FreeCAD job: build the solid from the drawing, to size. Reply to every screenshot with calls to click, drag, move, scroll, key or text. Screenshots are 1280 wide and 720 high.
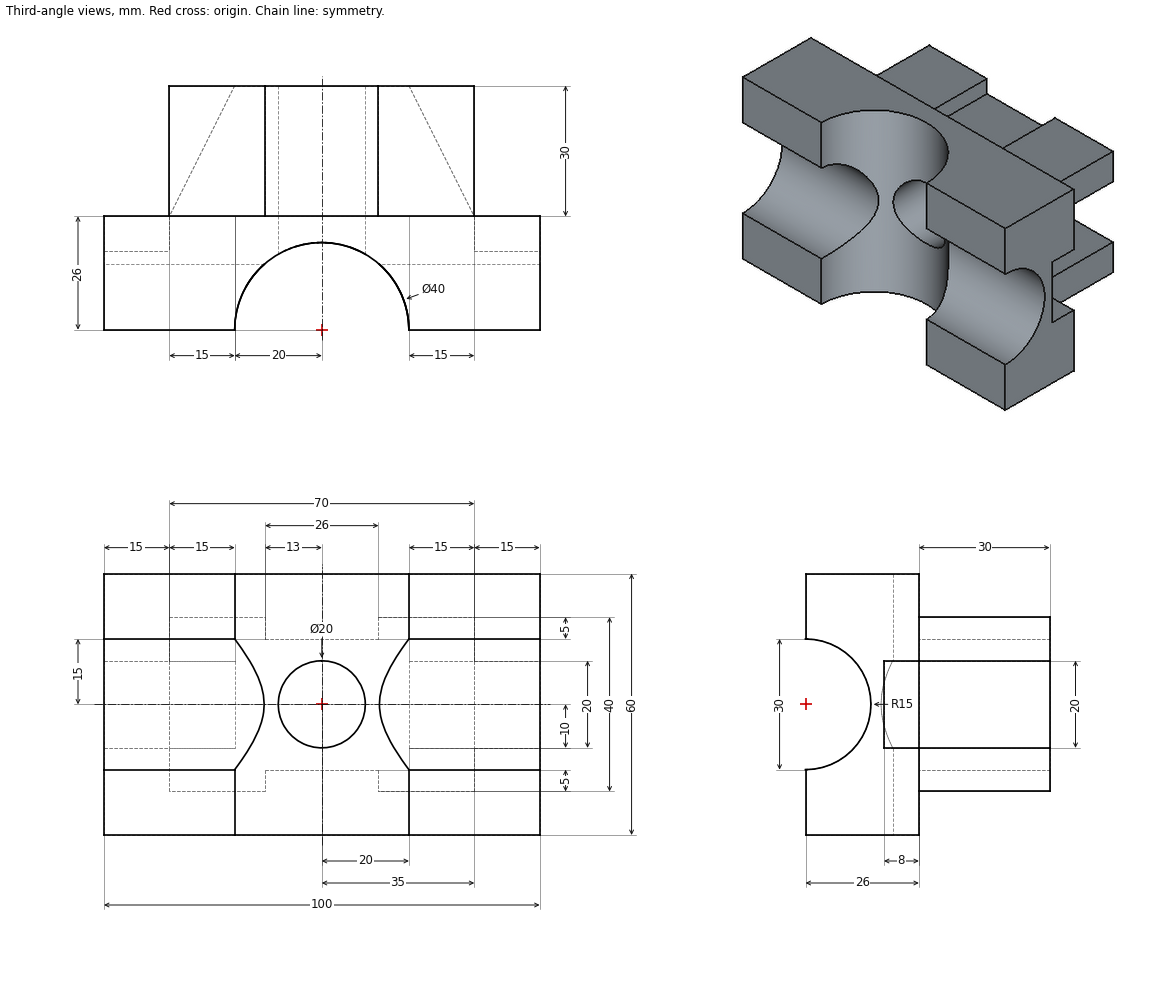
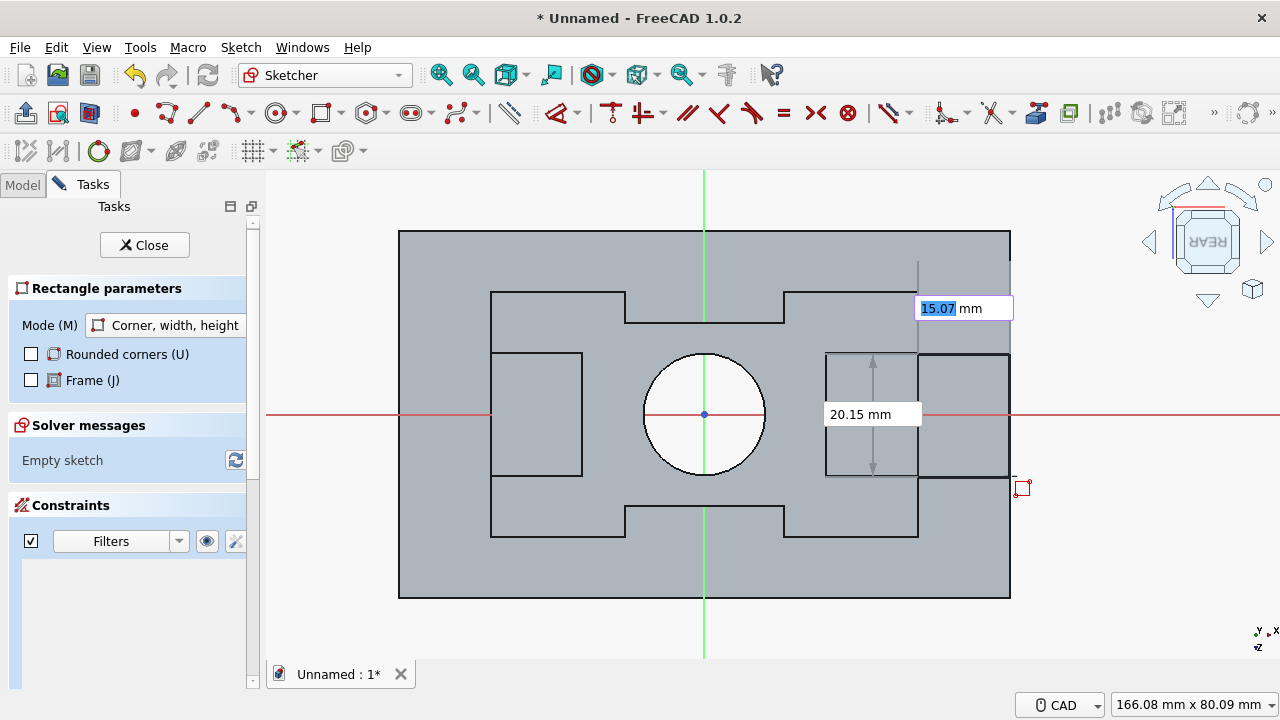
text(15)
key(Tab)
text(20)
key(Return)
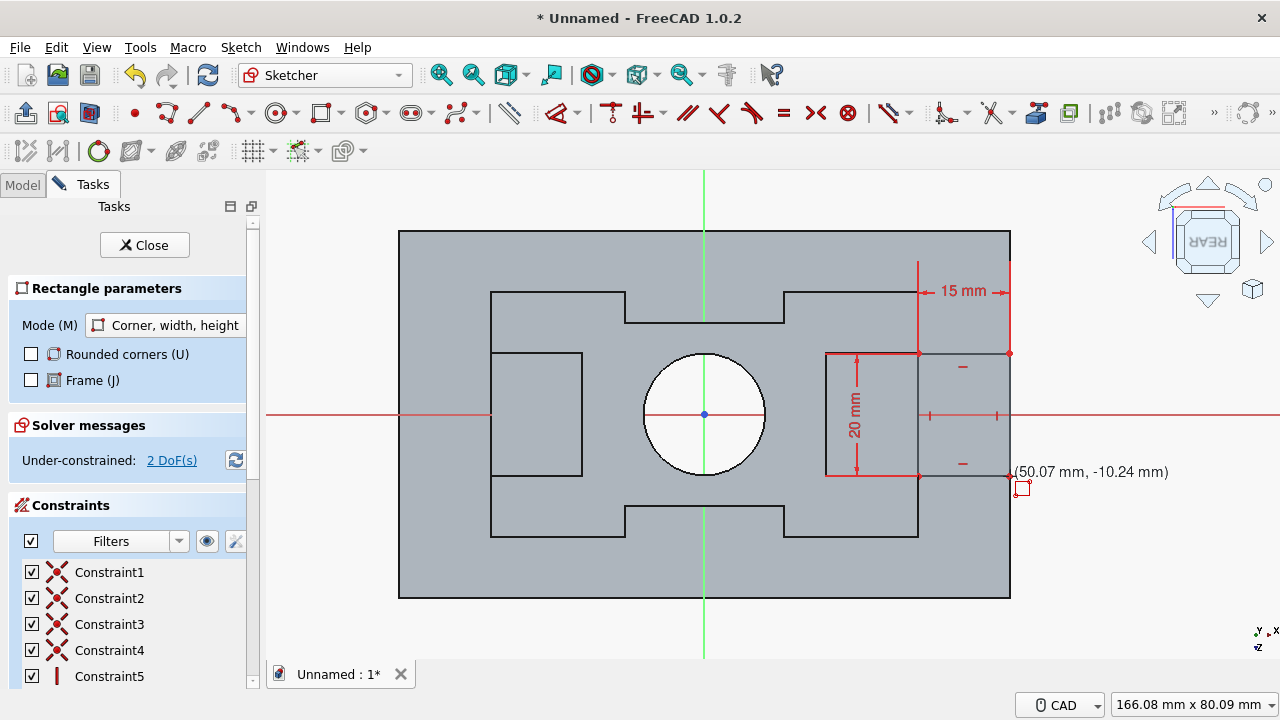
click(399, 353)
move(491, 476)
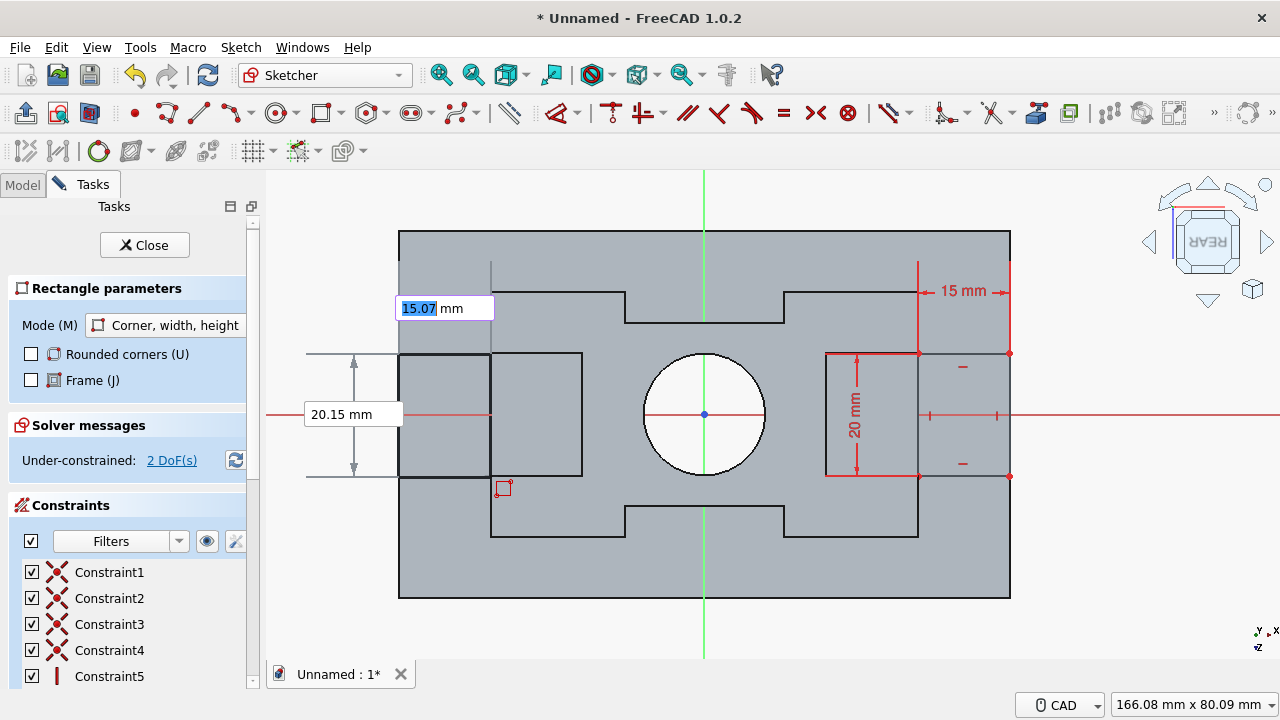
text(15)
key(Tab)
text(20)
key(Return)
key(Escape)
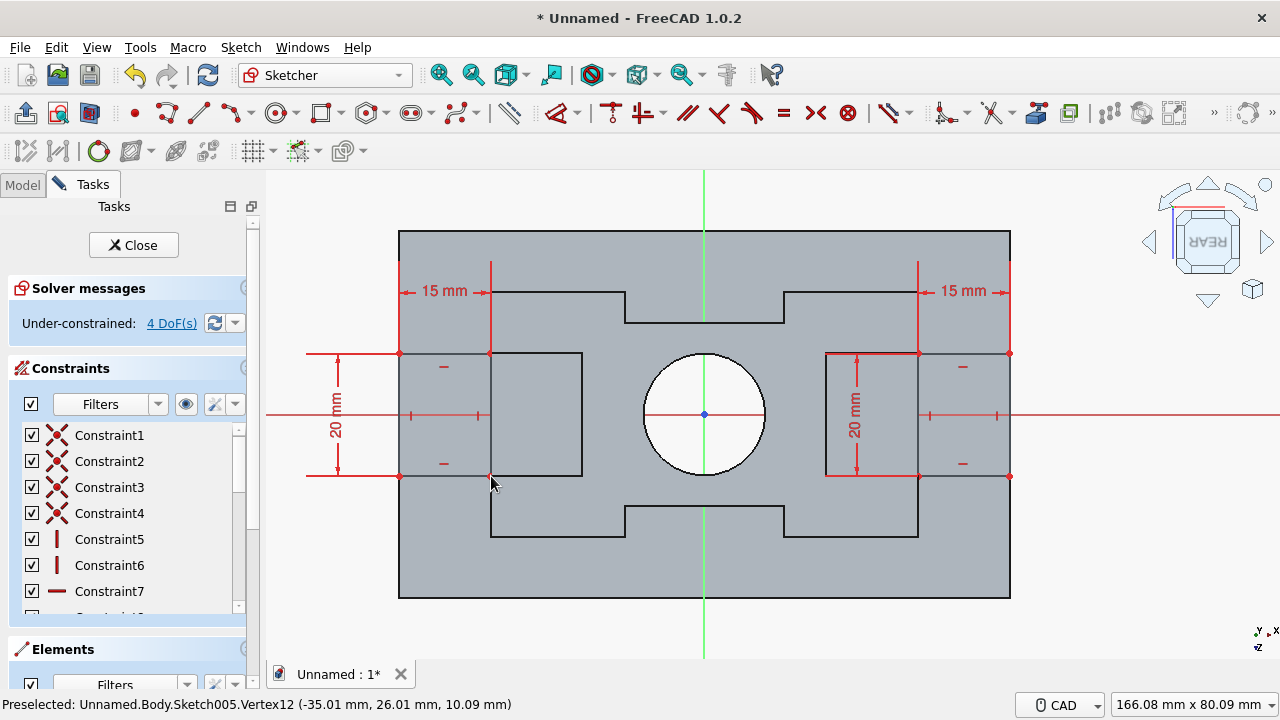
click(1010, 354)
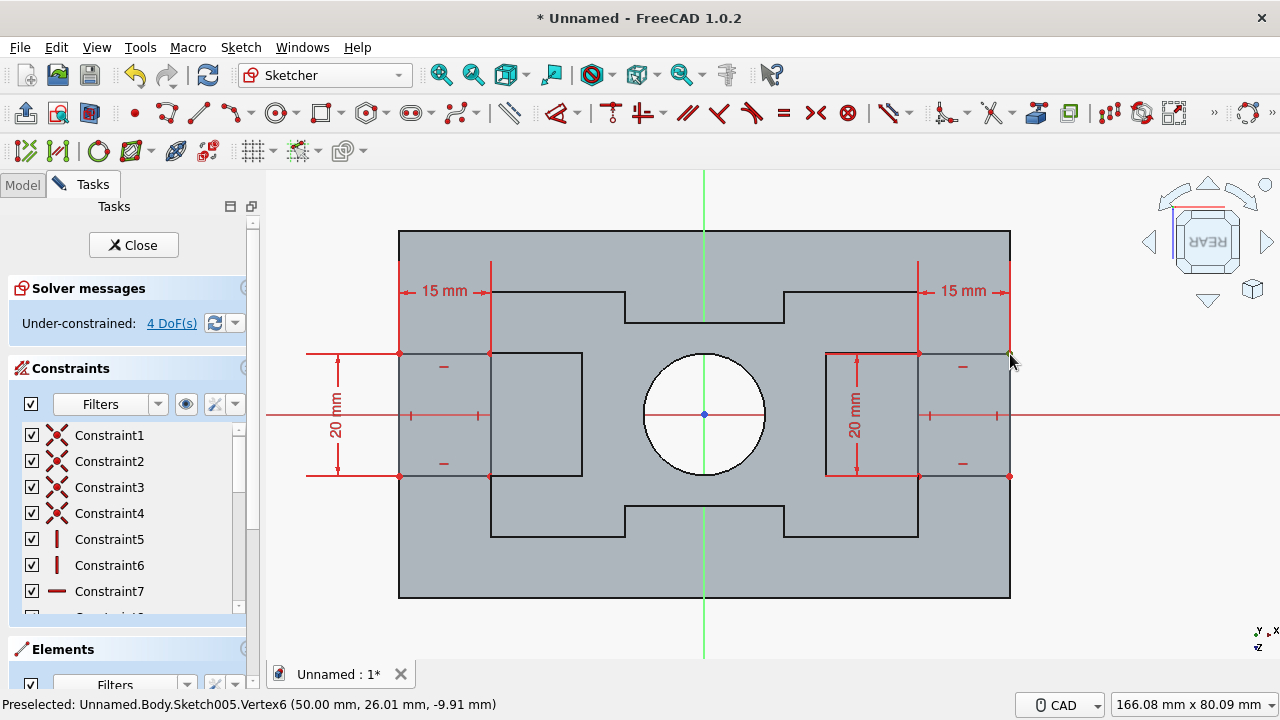
click(399, 354)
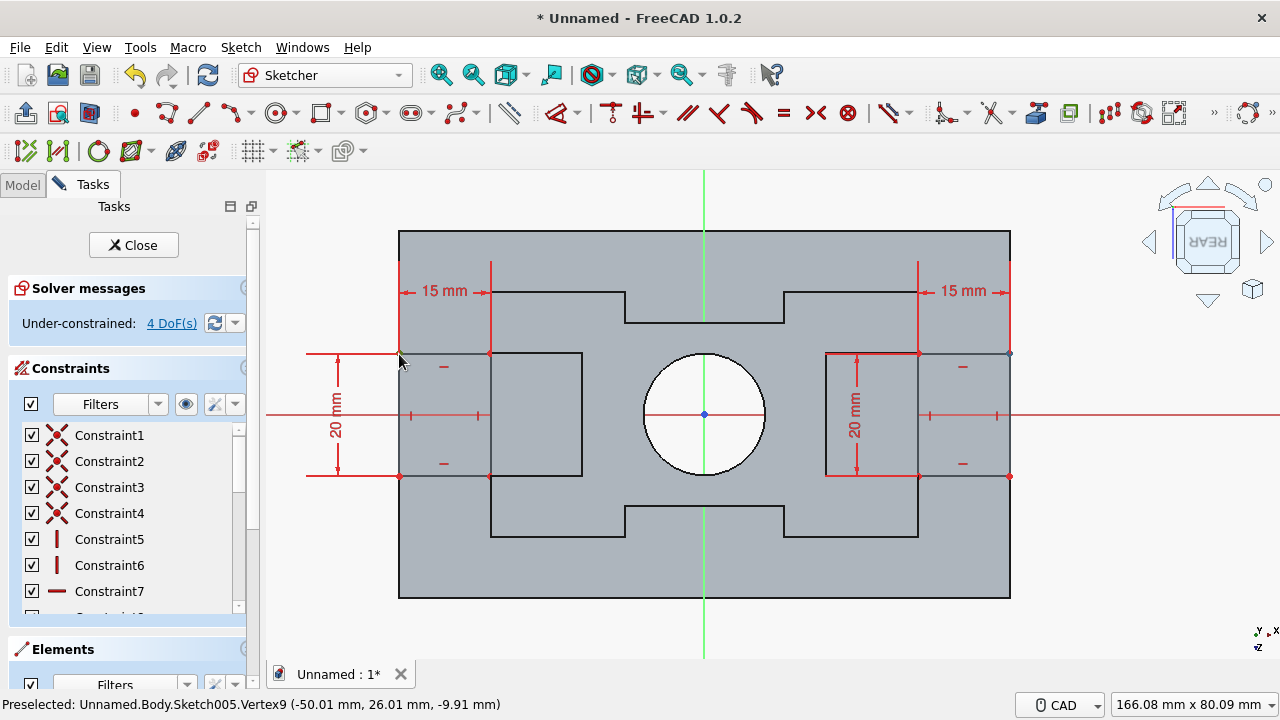
click(704, 600)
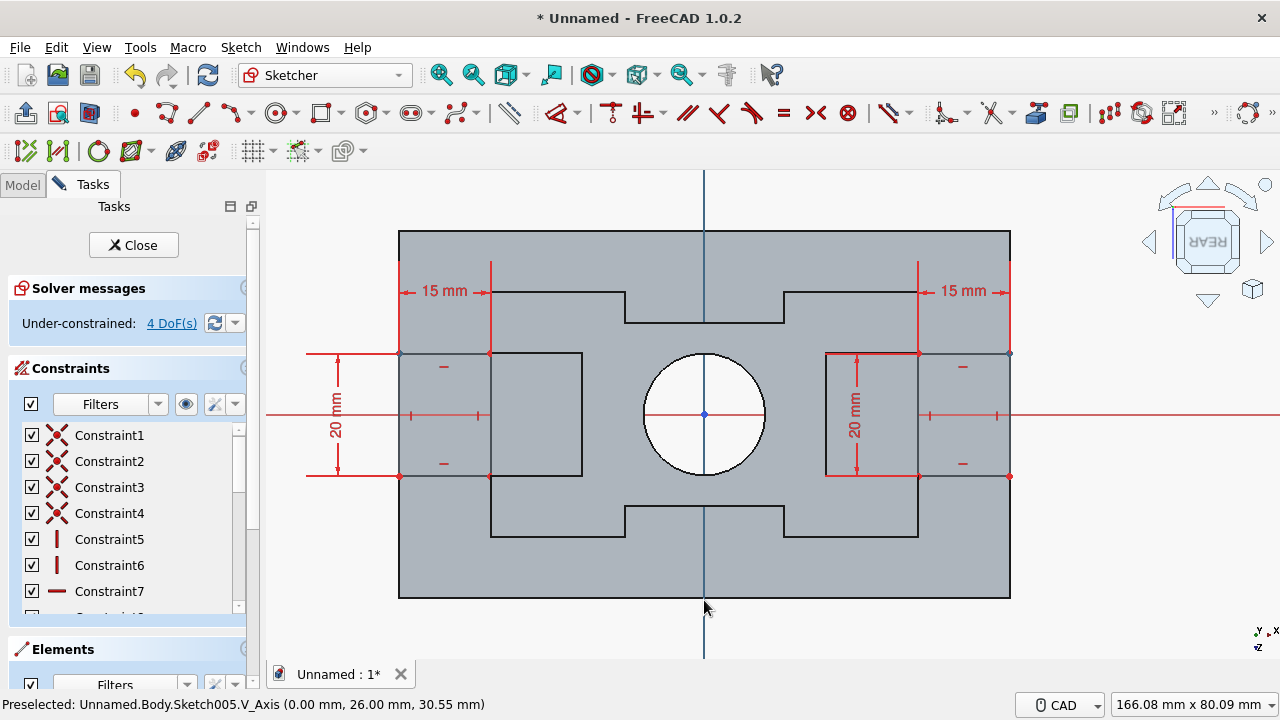
key(s)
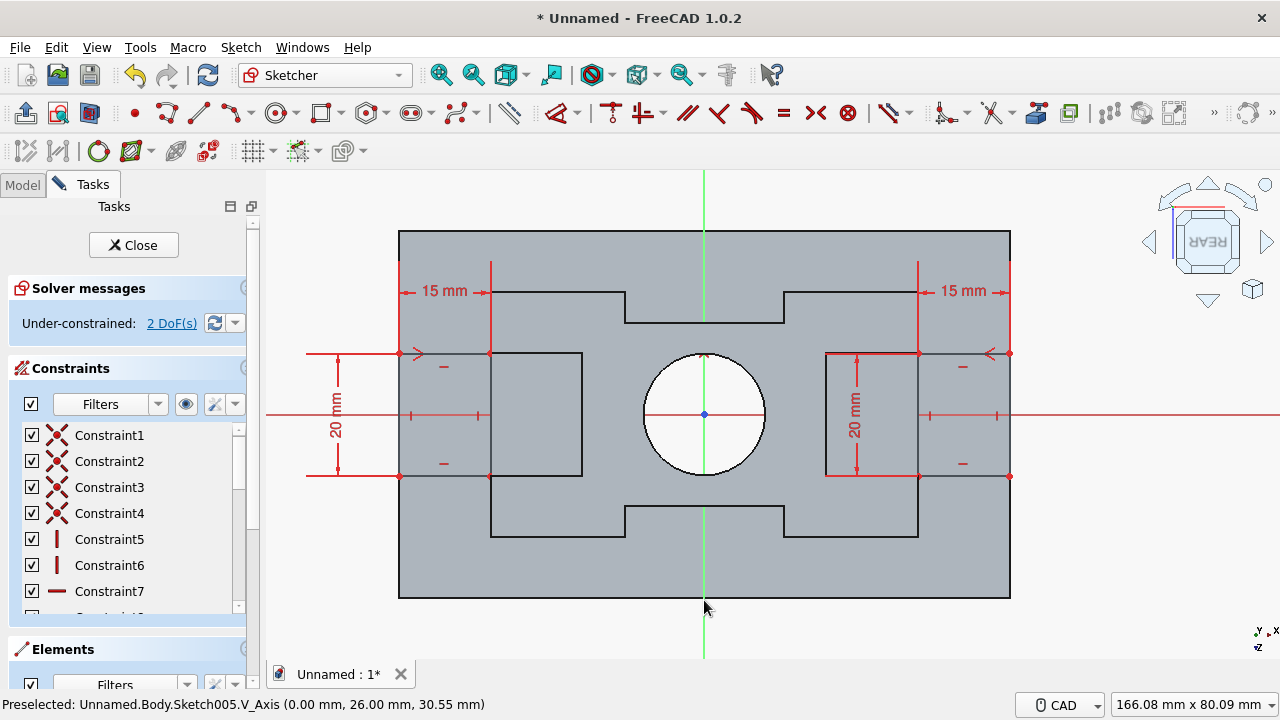
key(d)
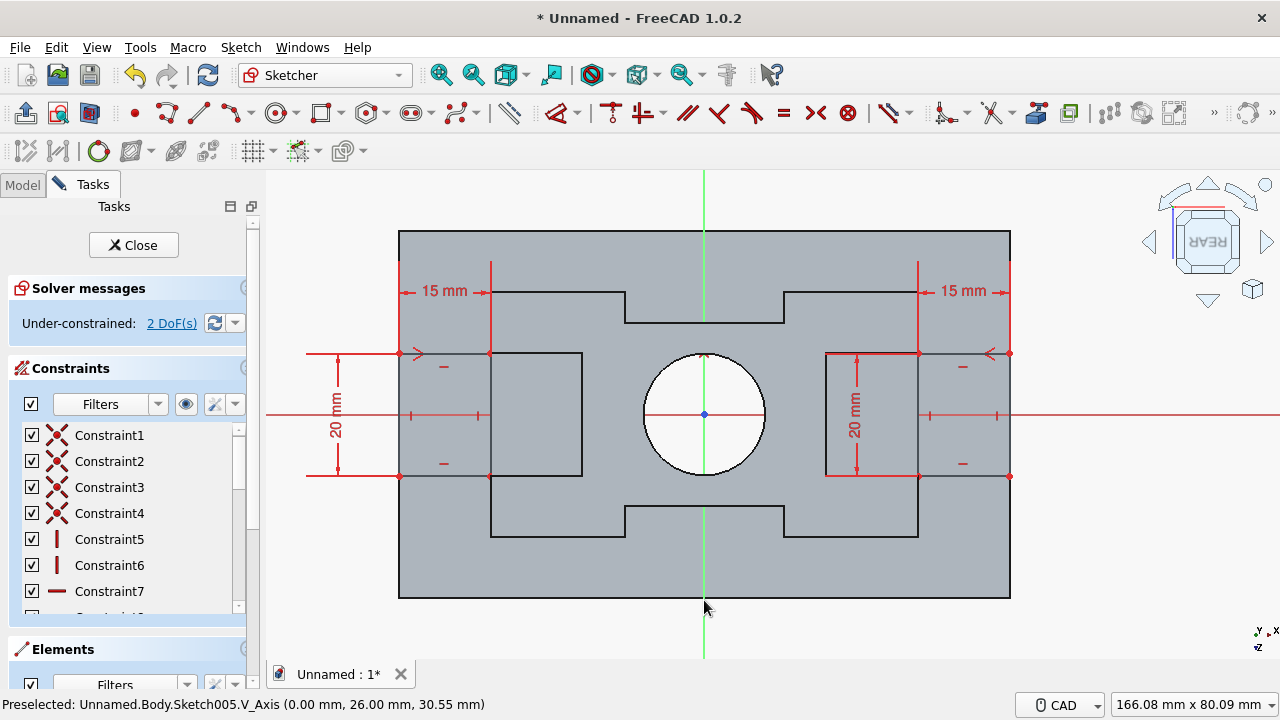
click(918, 354)
click(811, 320)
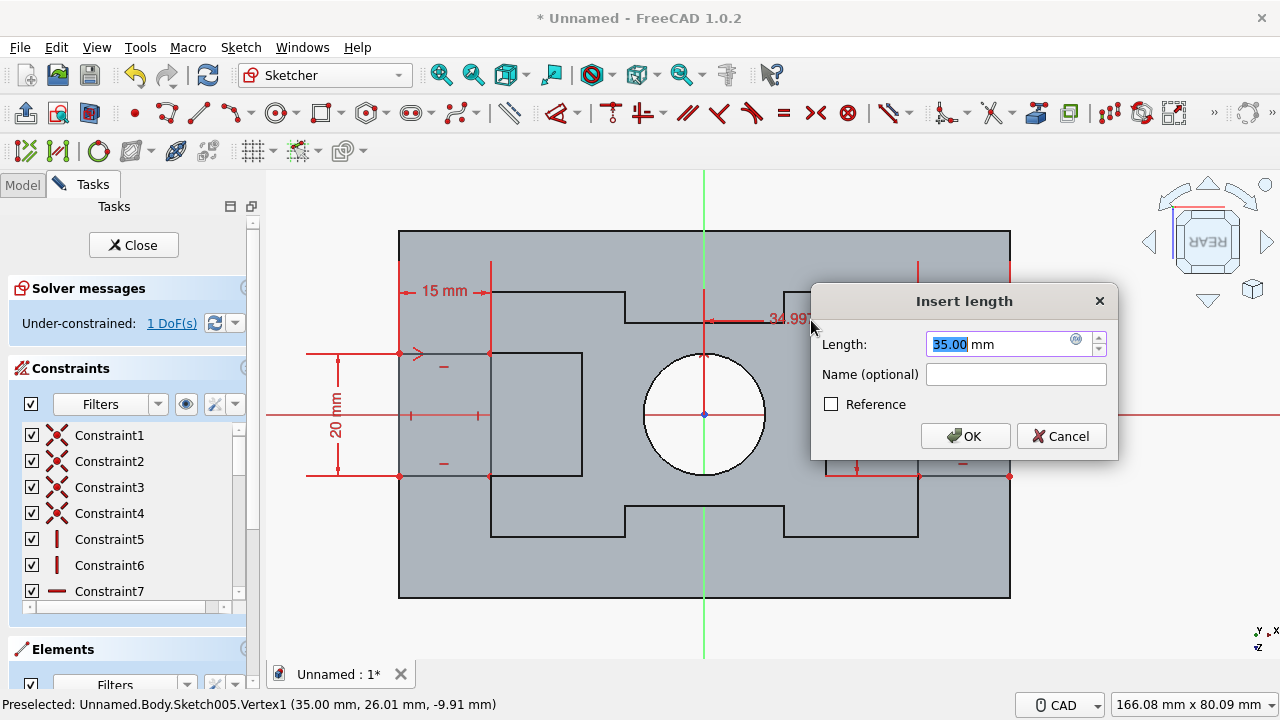
text(35)
key(Return)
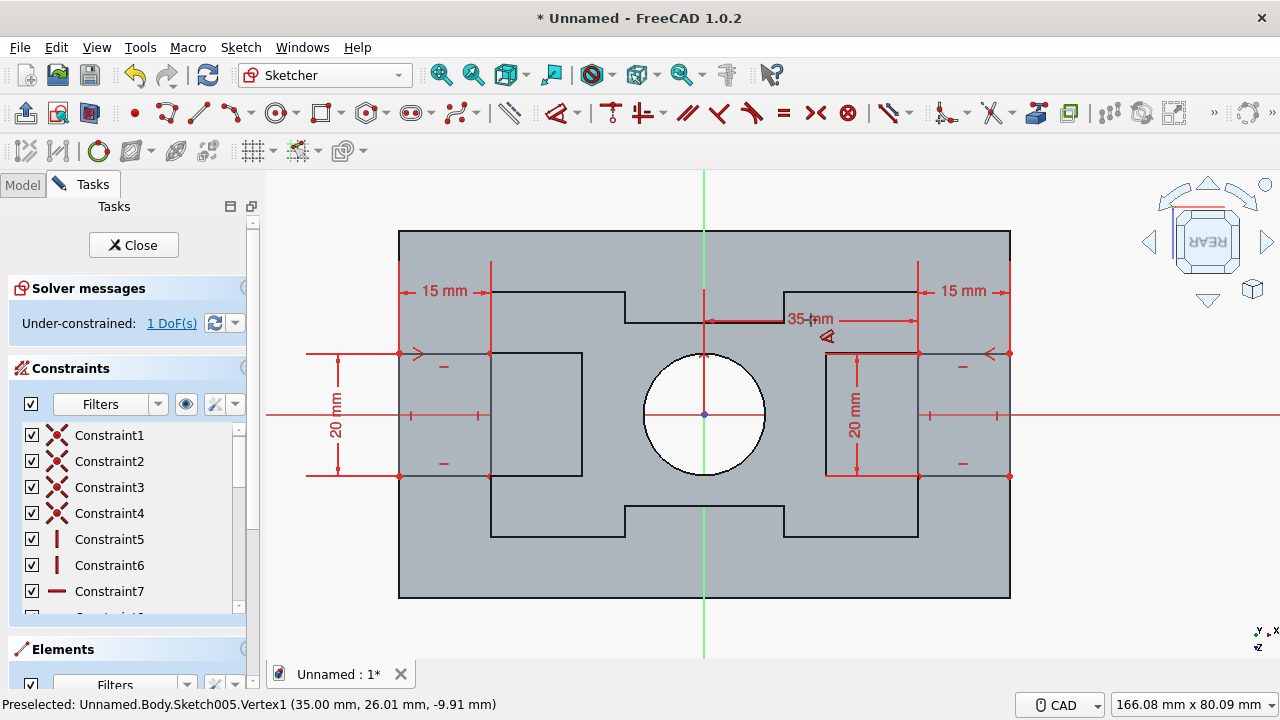
click(918, 354)
click(952, 384)